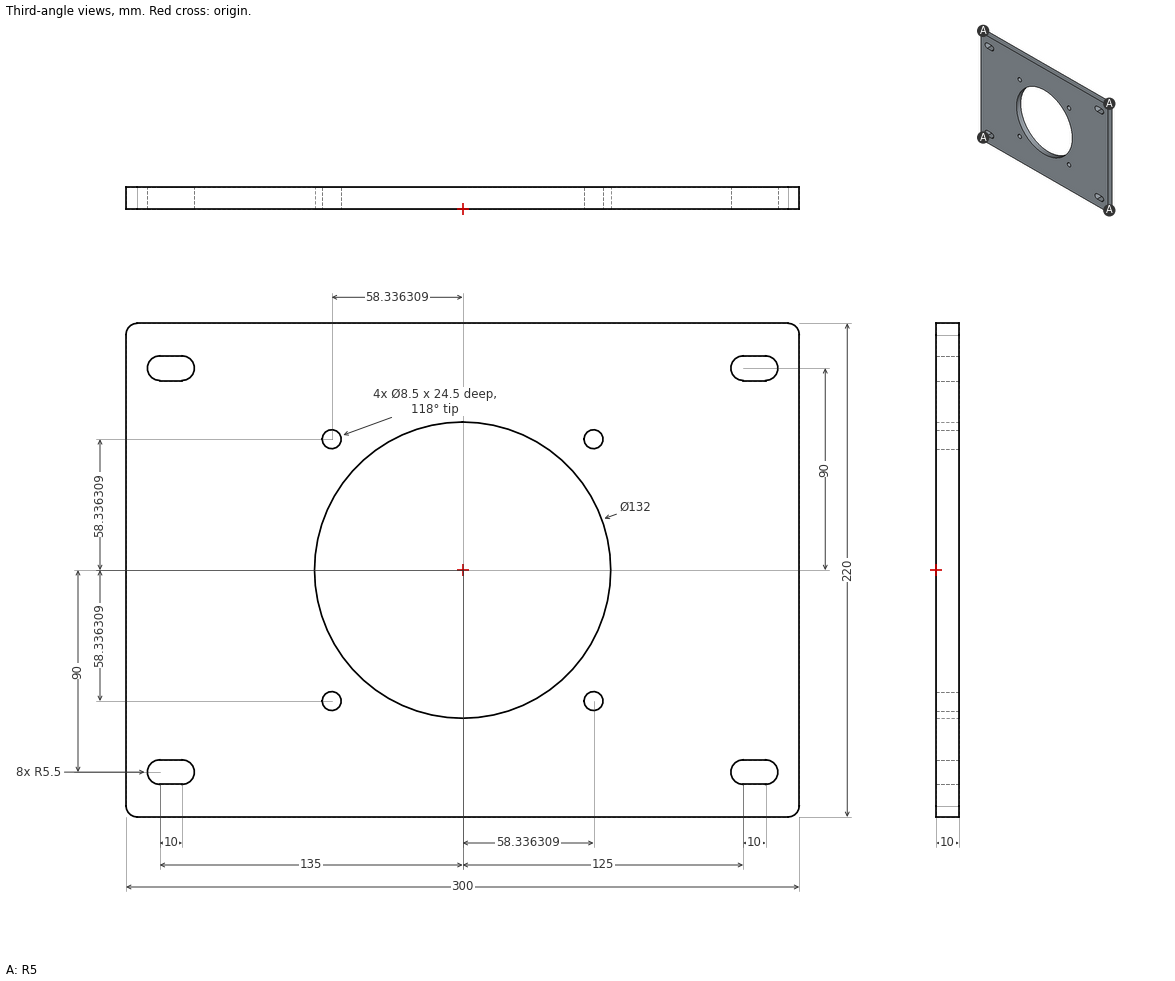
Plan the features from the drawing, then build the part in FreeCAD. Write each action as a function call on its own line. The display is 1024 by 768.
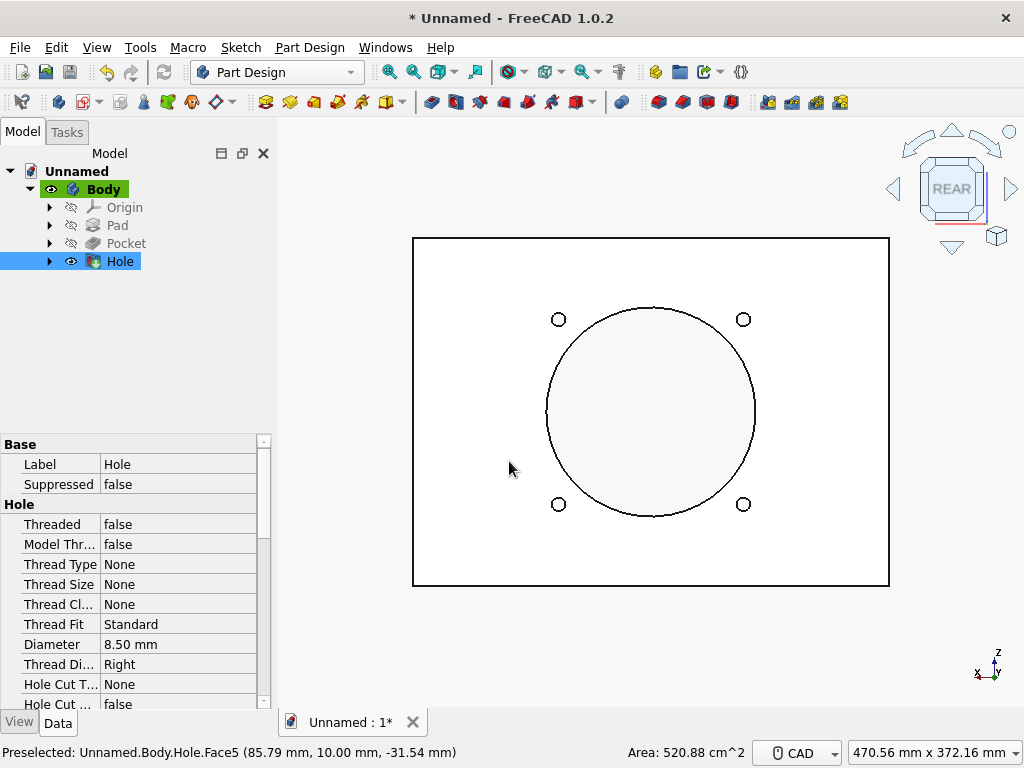
click(84, 102)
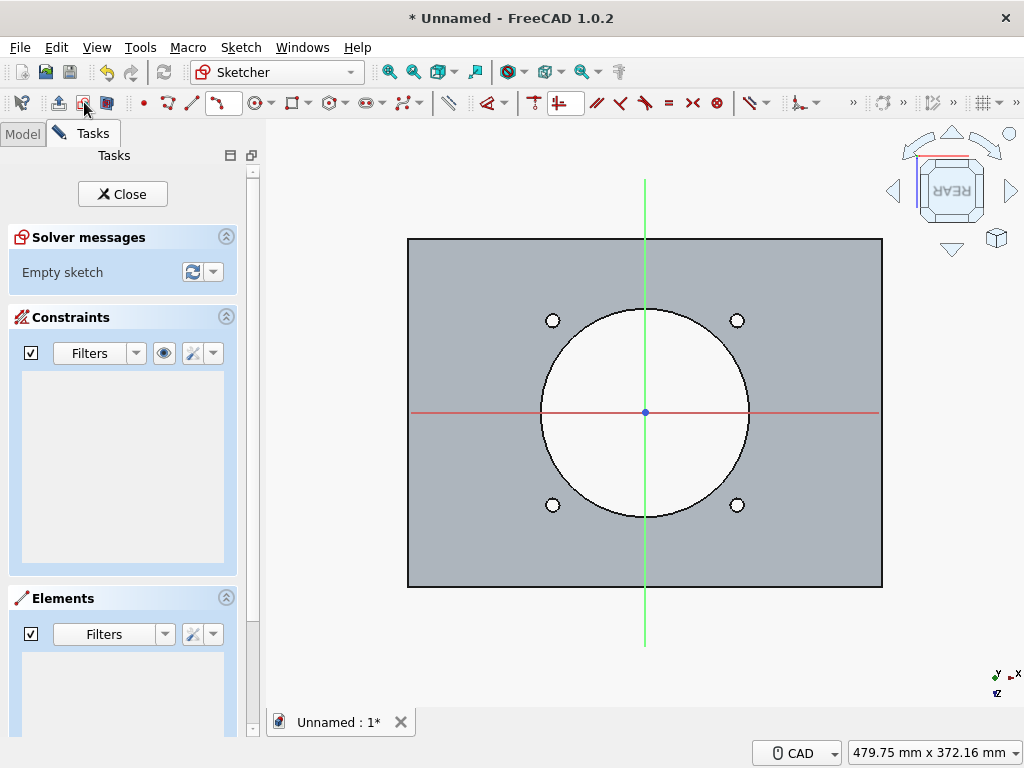
scroll(294, 413, down, 1)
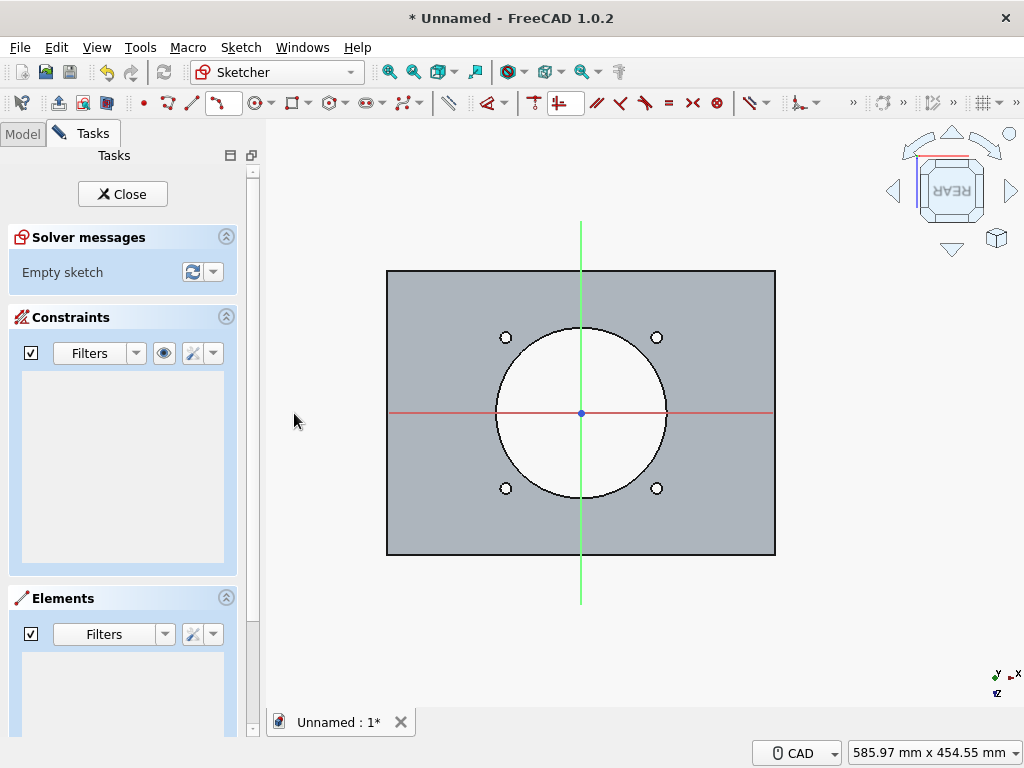
key(g)
key(s)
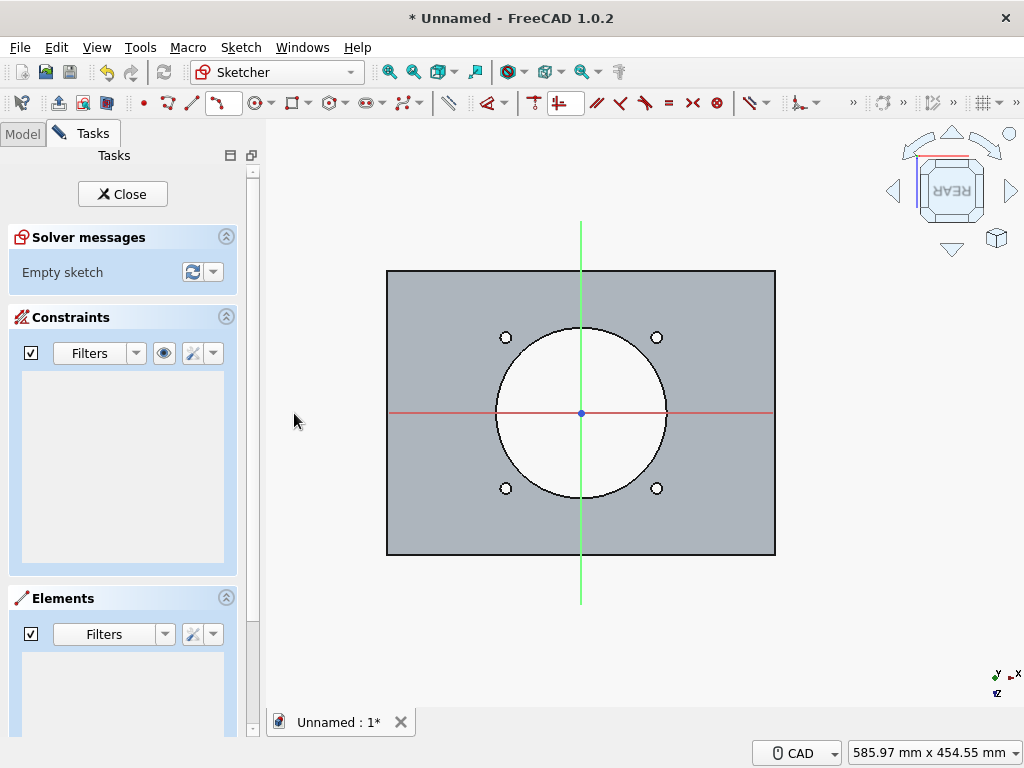
scroll(407, 297, up, 6)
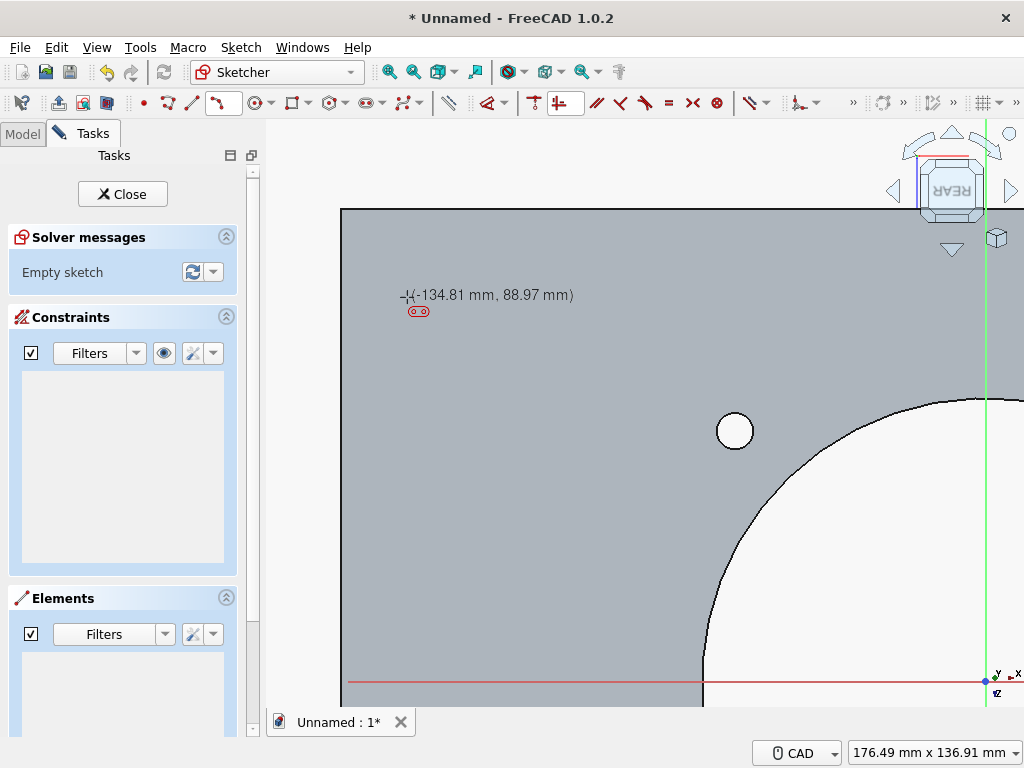
click(406, 295)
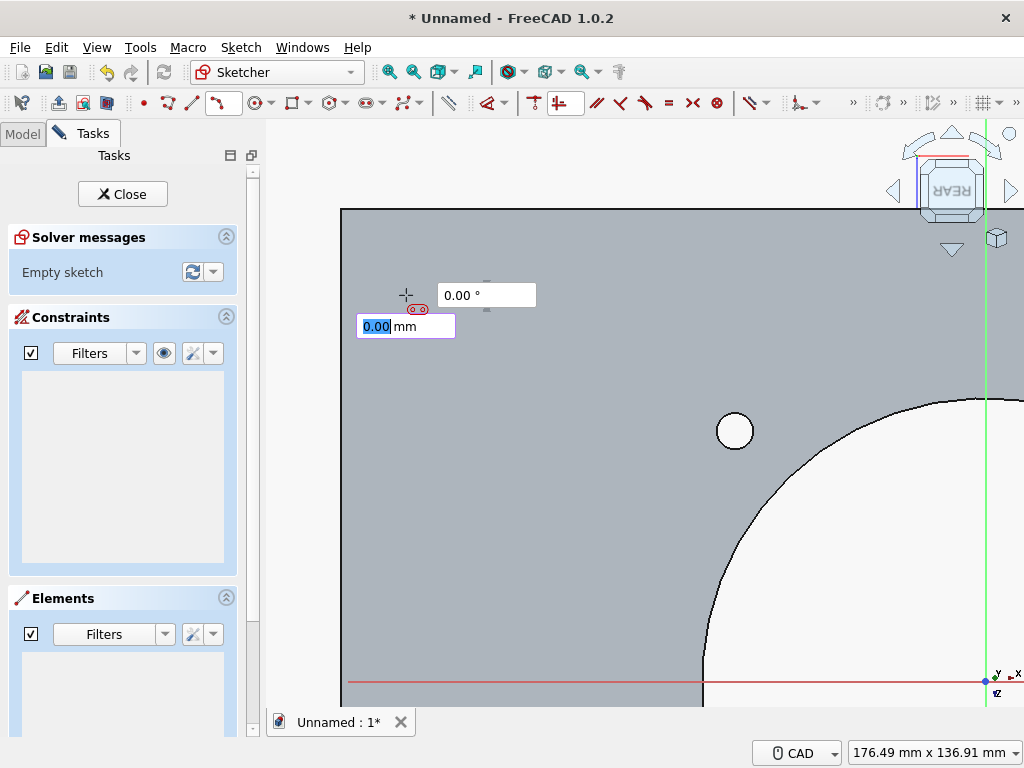
click(449, 295)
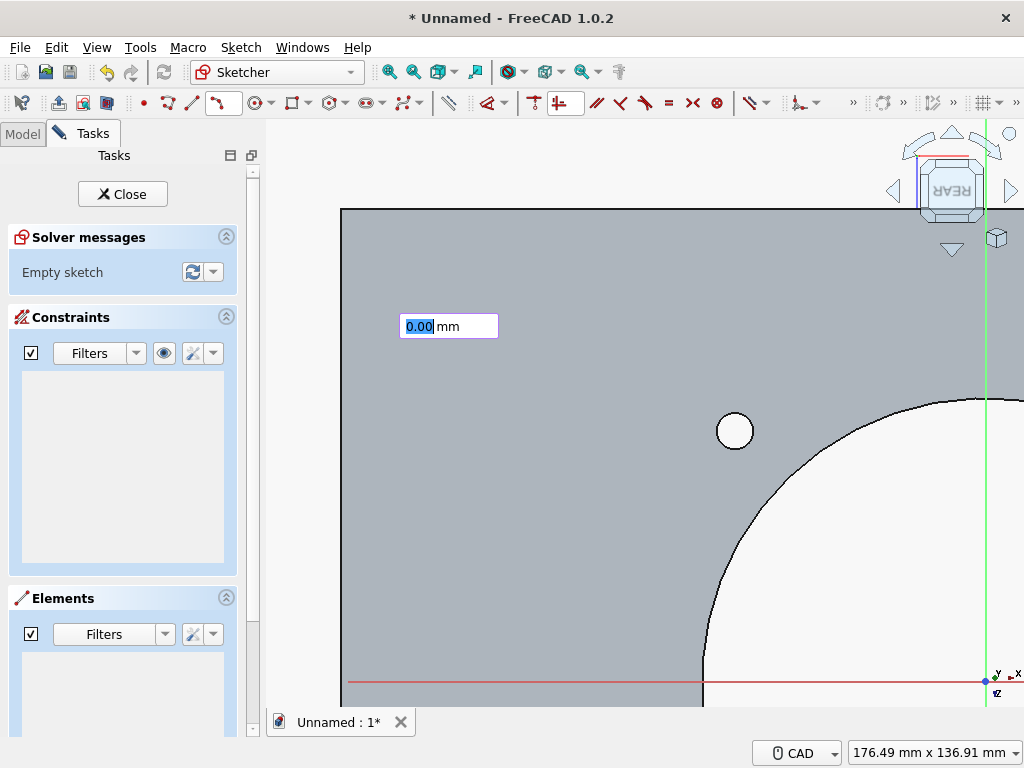
click(427, 272)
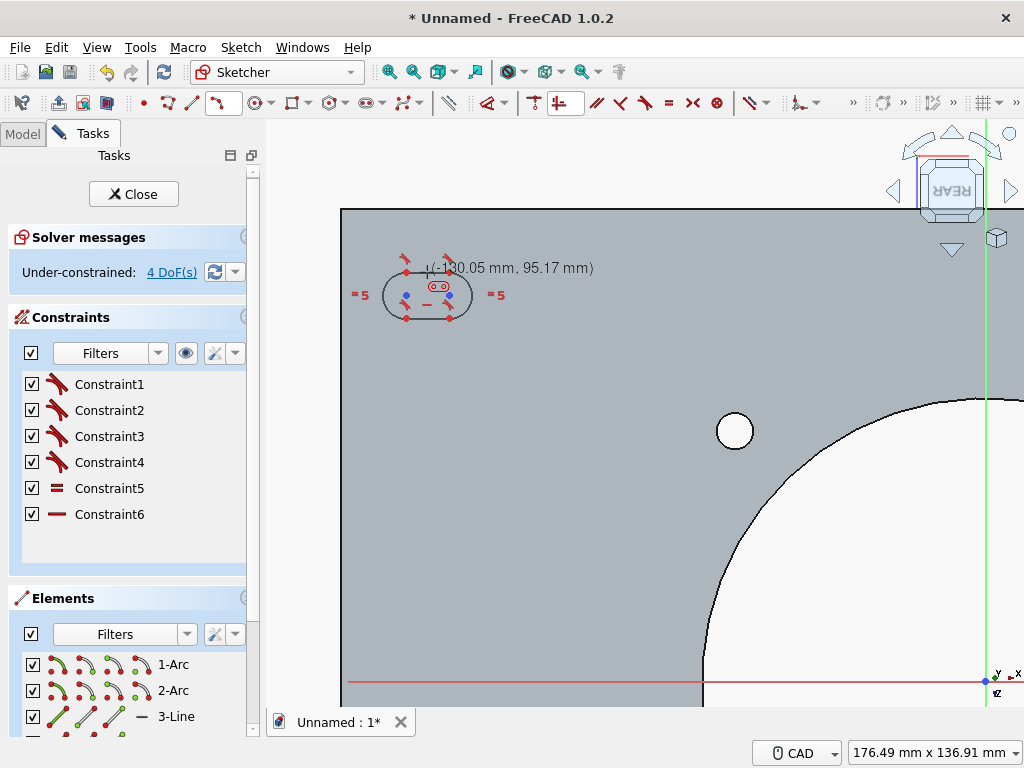
scroll(400, 297, down, 6)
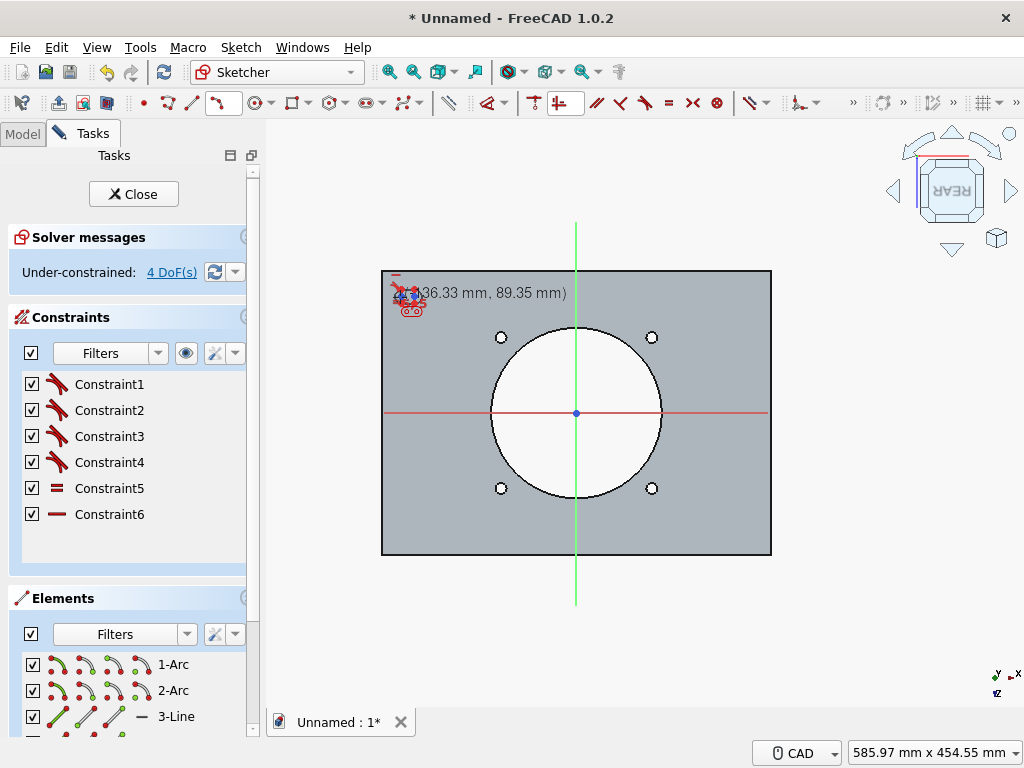
scroll(738, 297, up, 6)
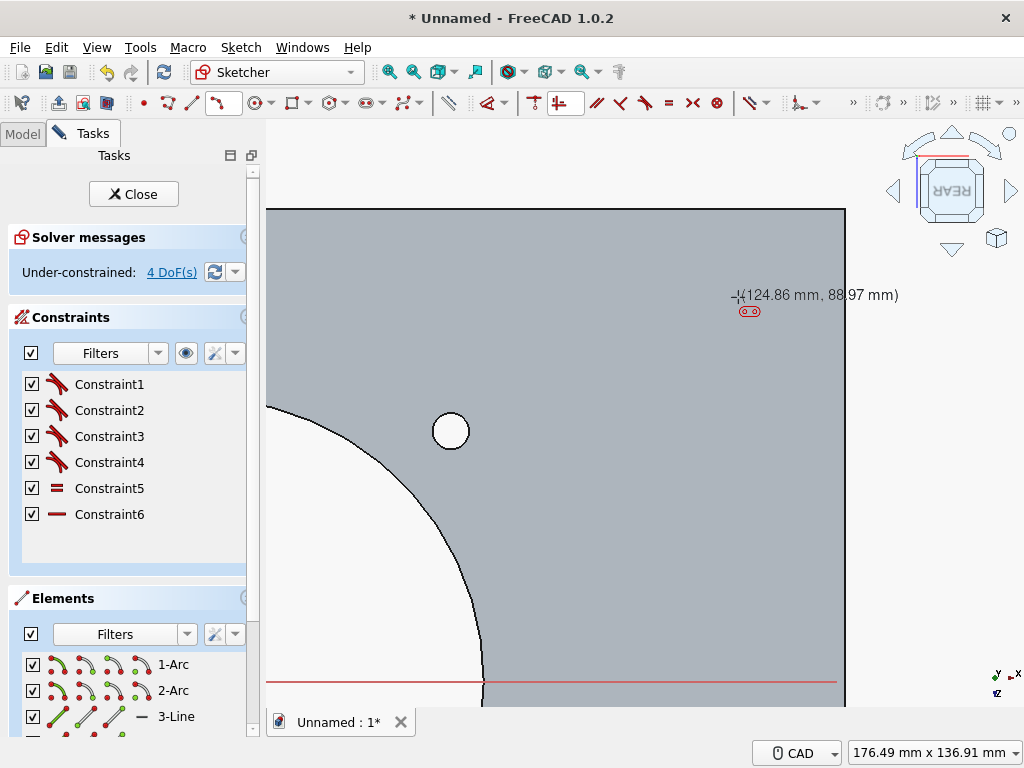
click(737, 295)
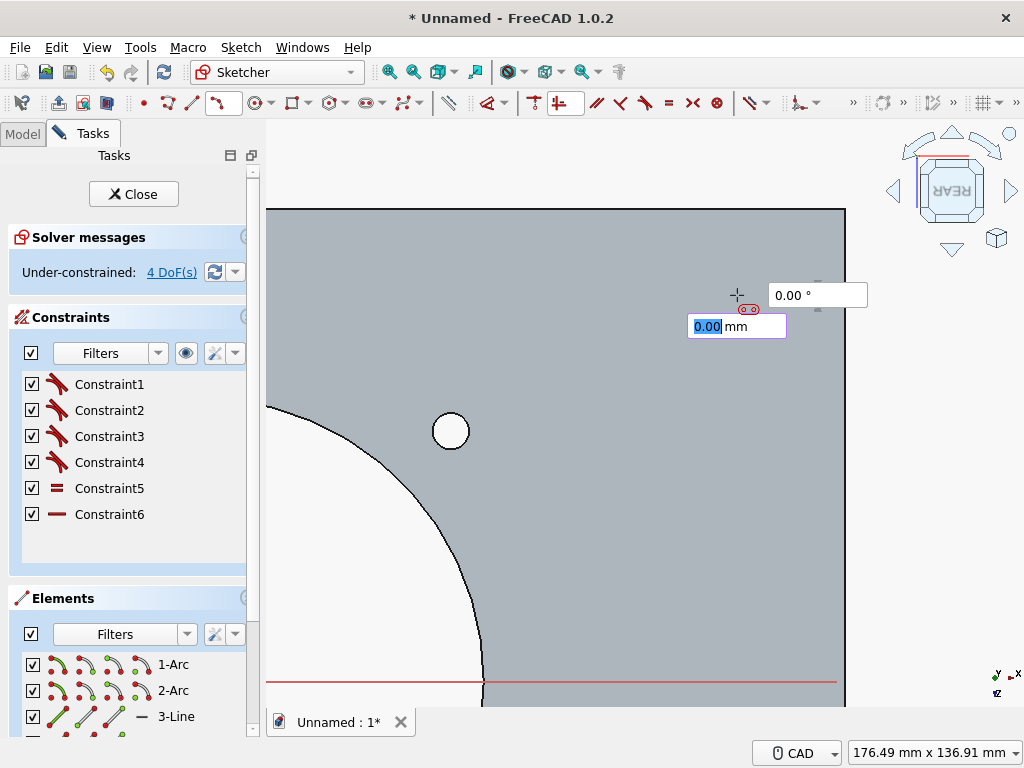
click(780, 295)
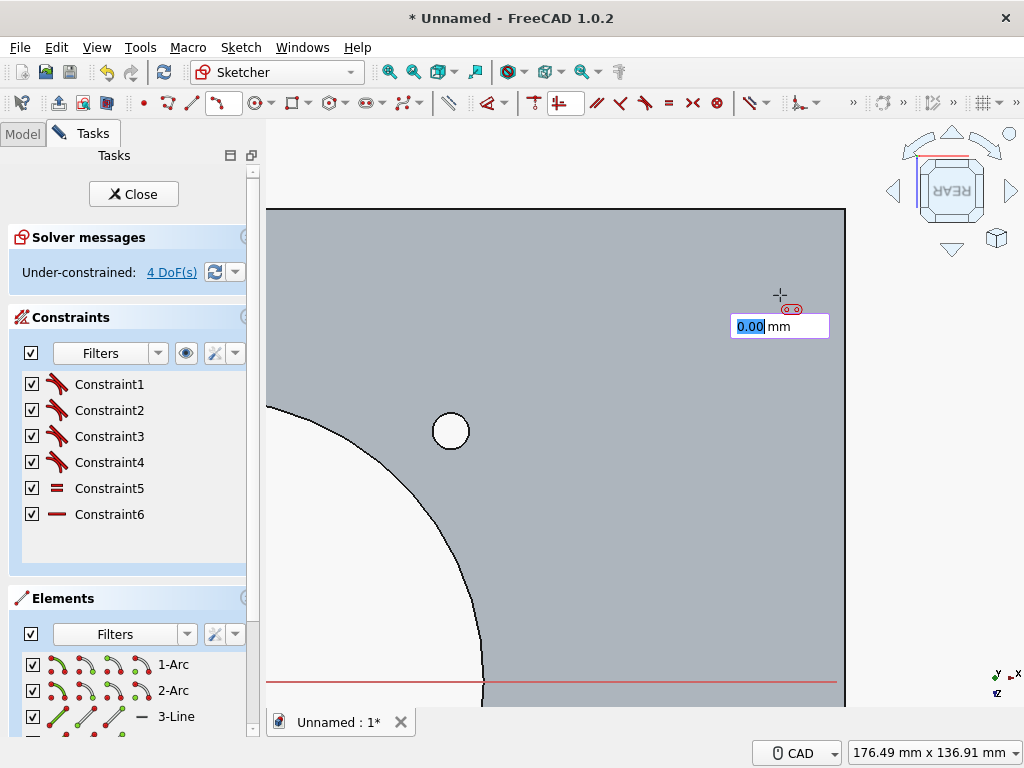
click(759, 272)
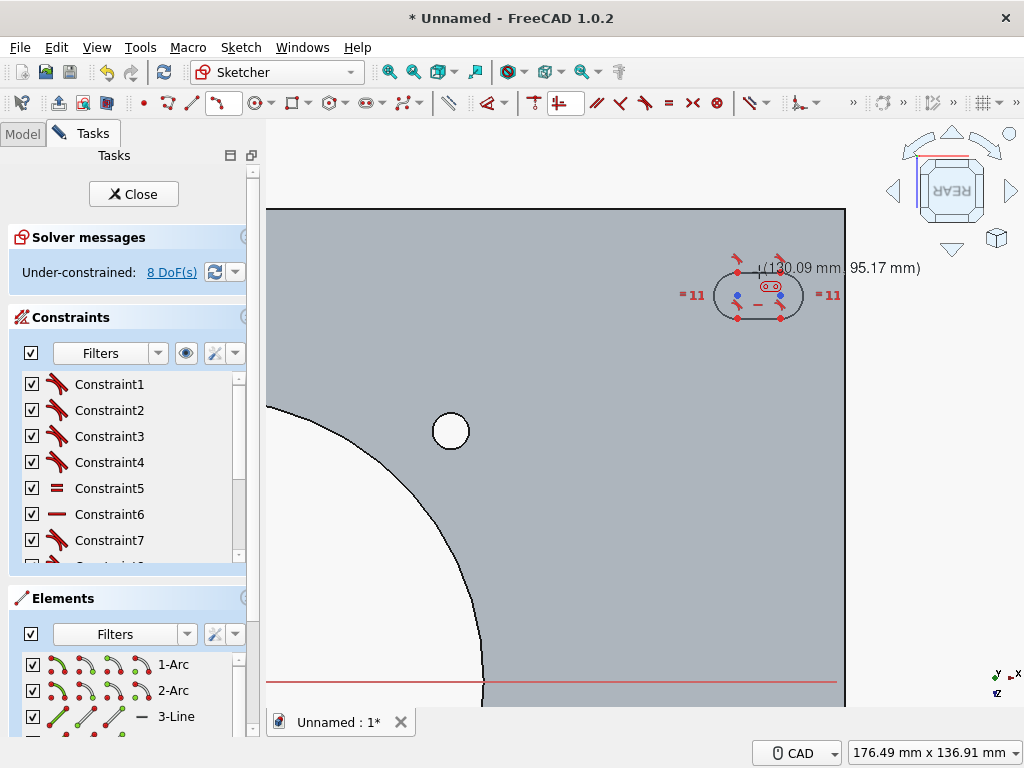
scroll(739, 297, down, 6)